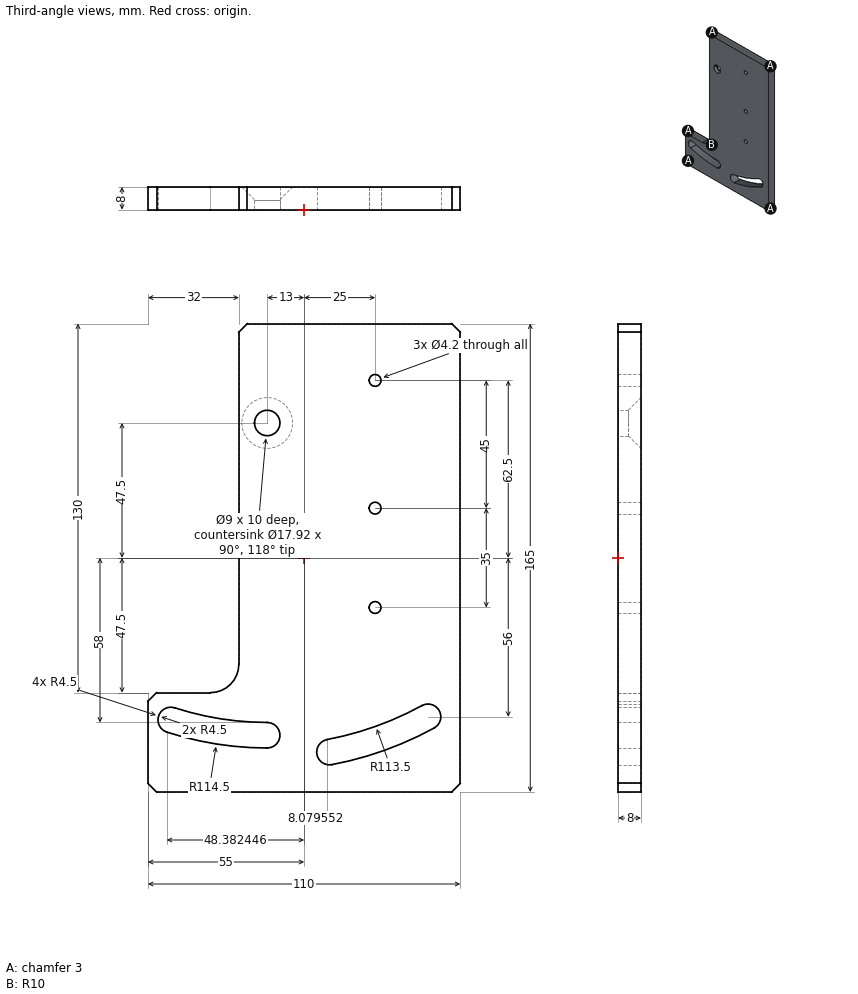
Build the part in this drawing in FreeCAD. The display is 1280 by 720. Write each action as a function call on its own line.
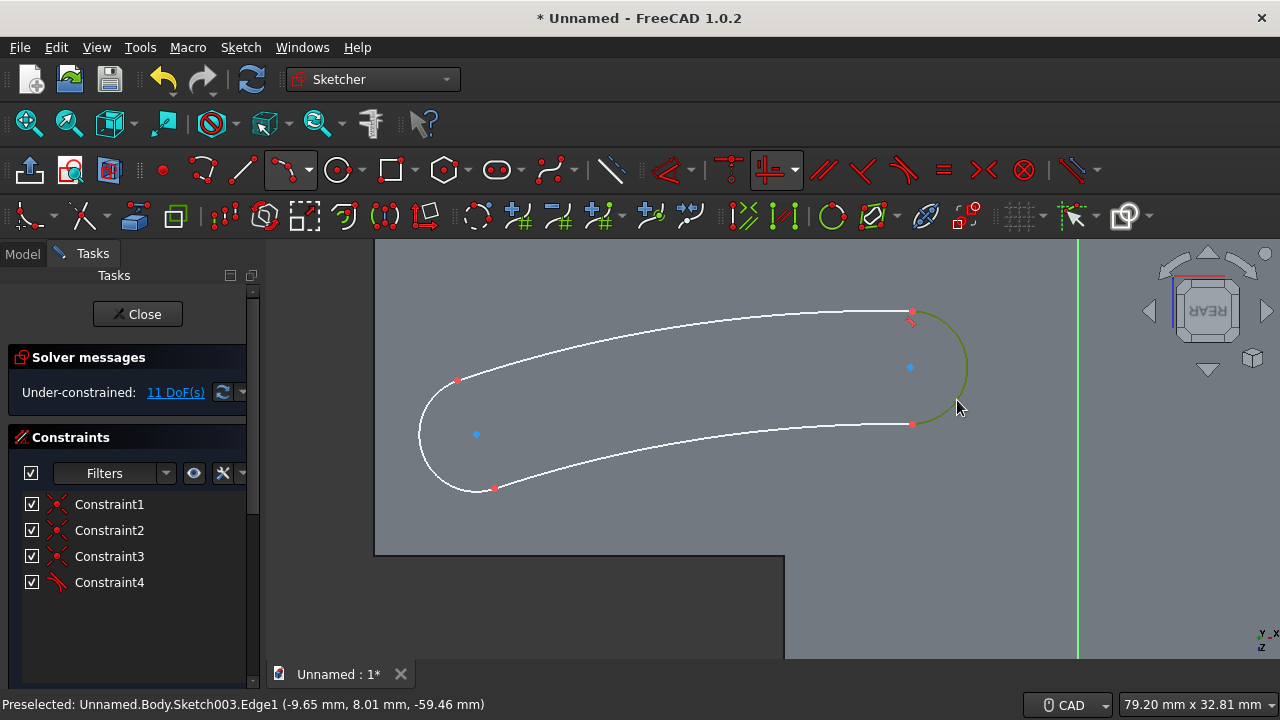
click(785, 429)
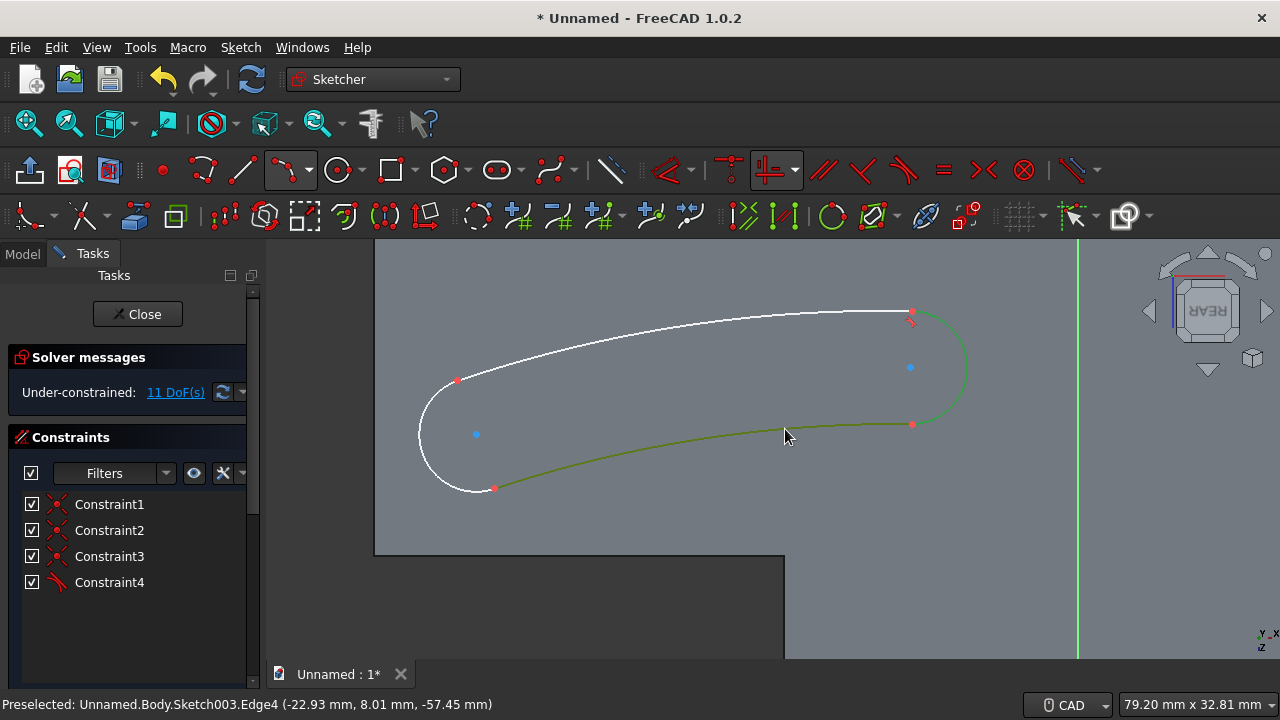
click(904, 170)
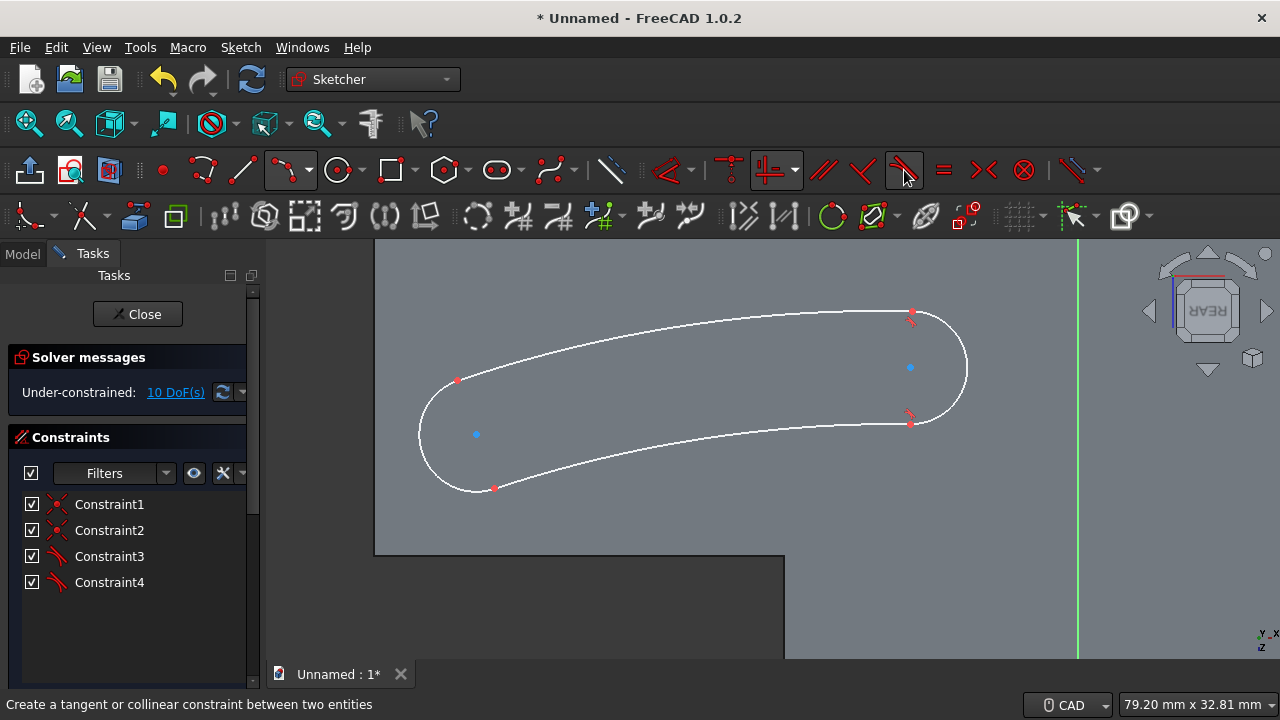
click(774, 315)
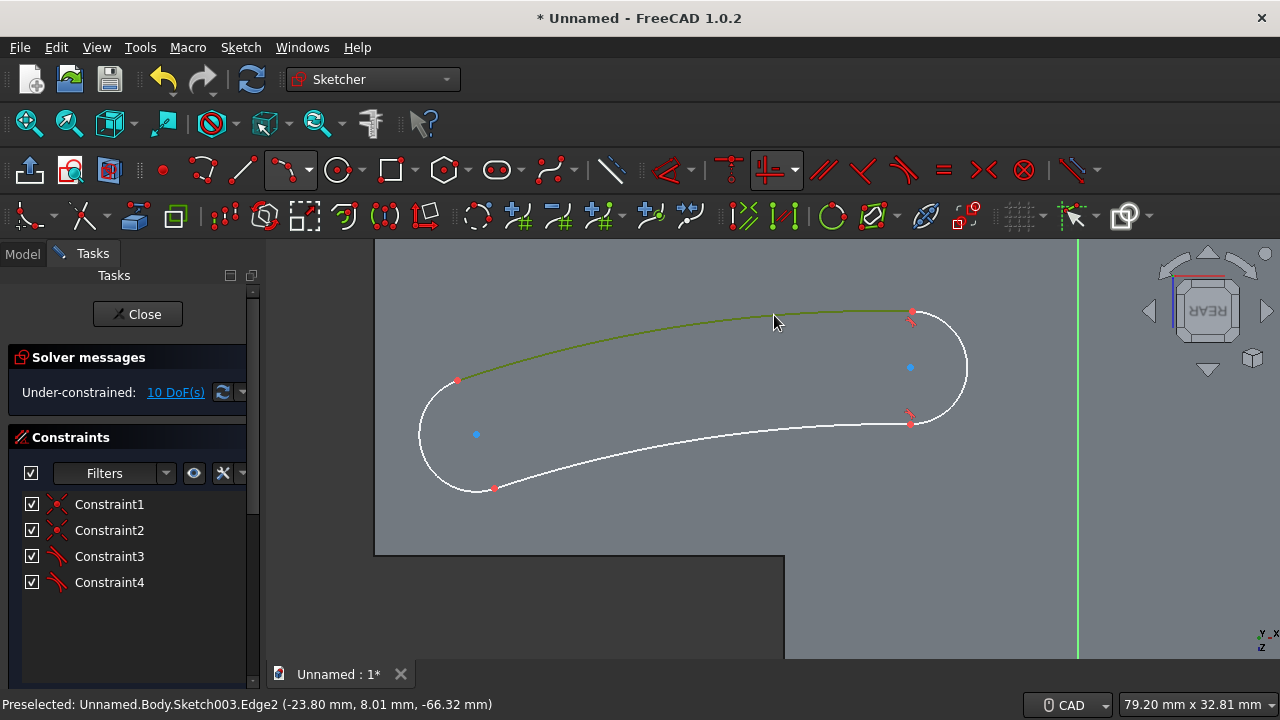
click(422, 418)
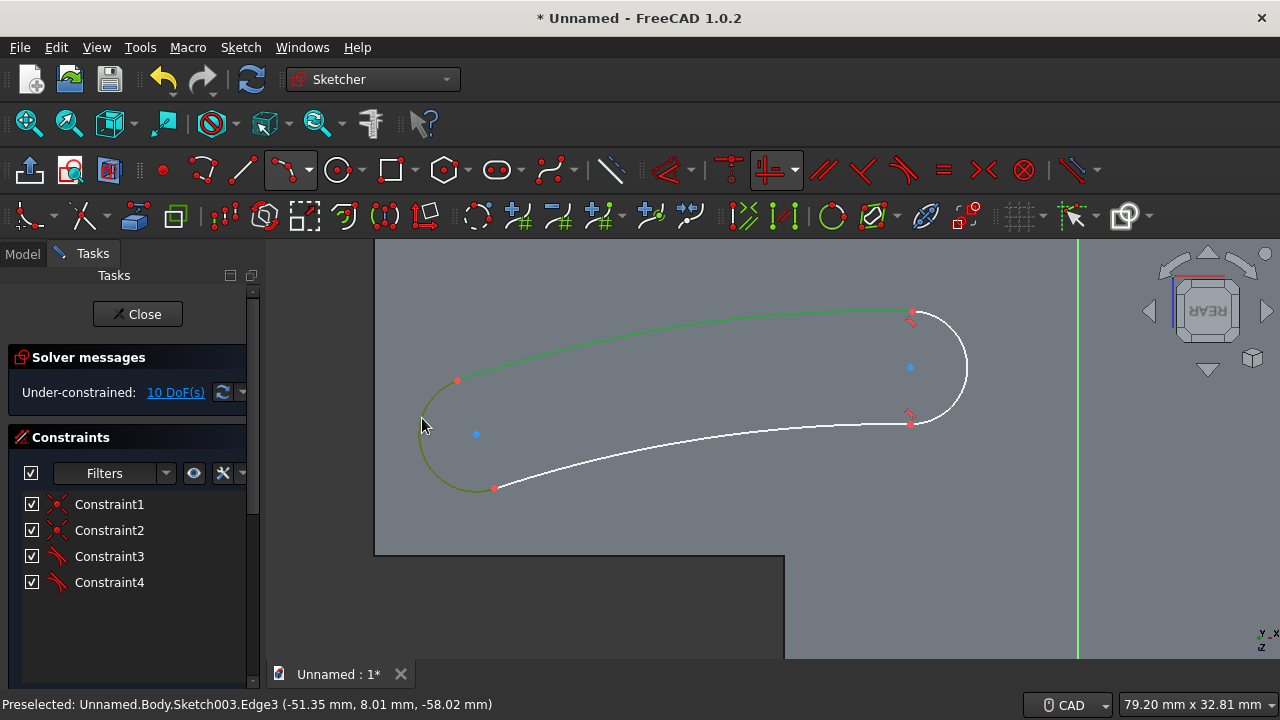
click(904, 170)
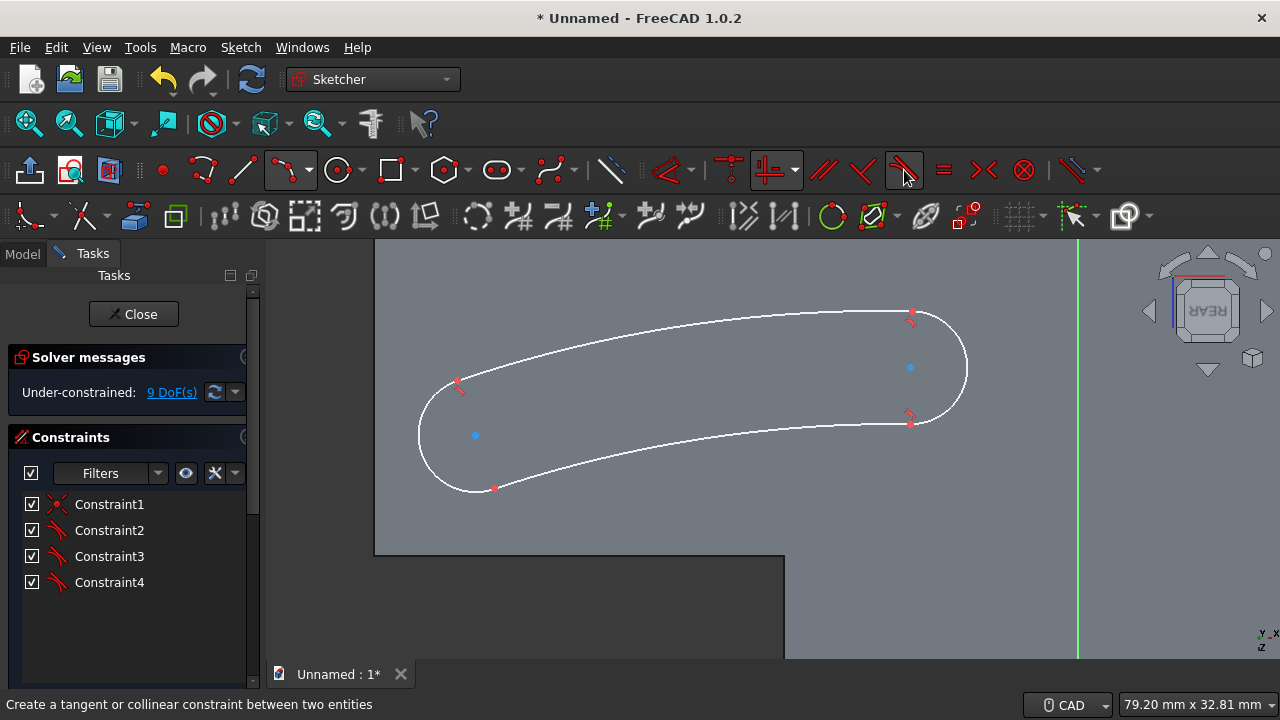
click(421, 418)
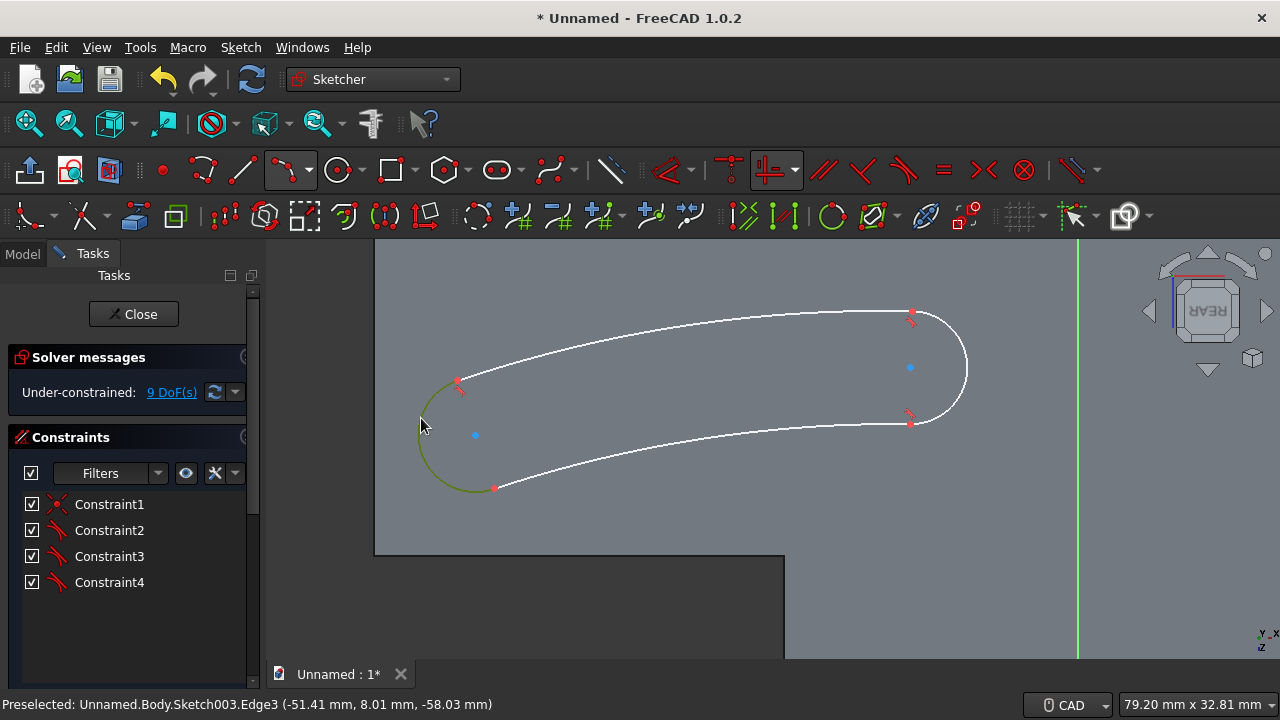
click(783, 429)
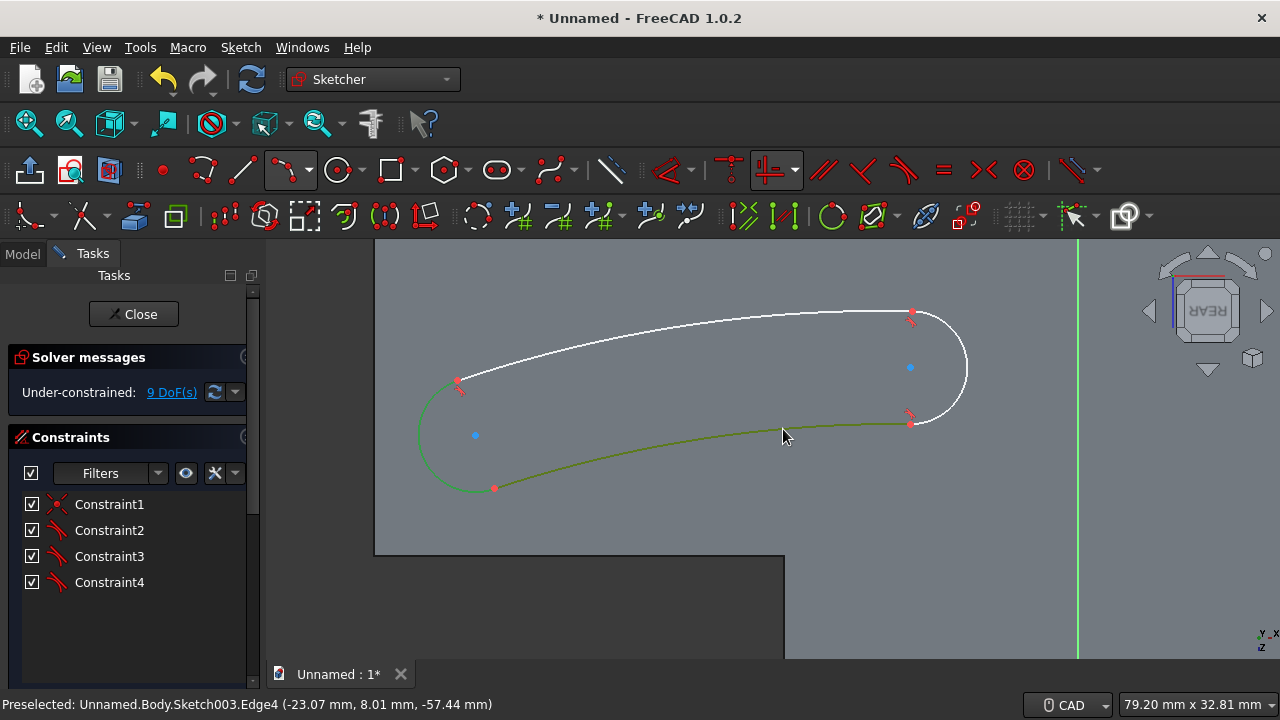
click(904, 170)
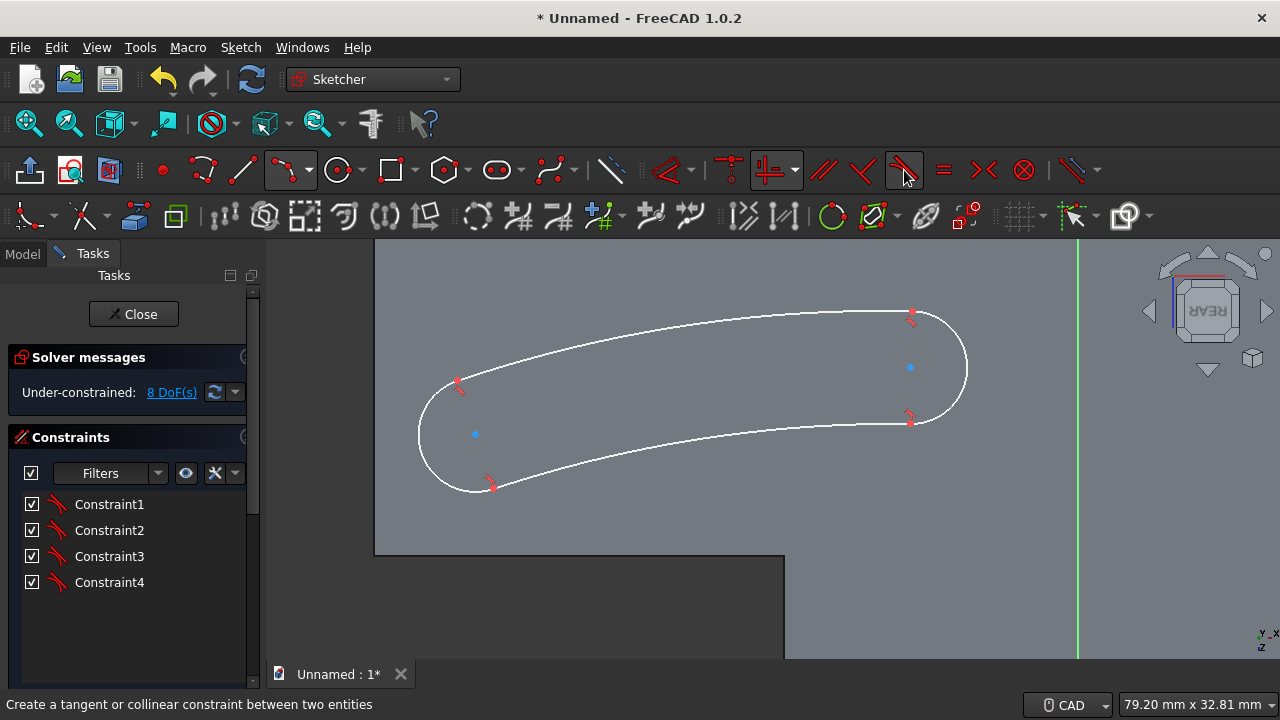
click(774, 315)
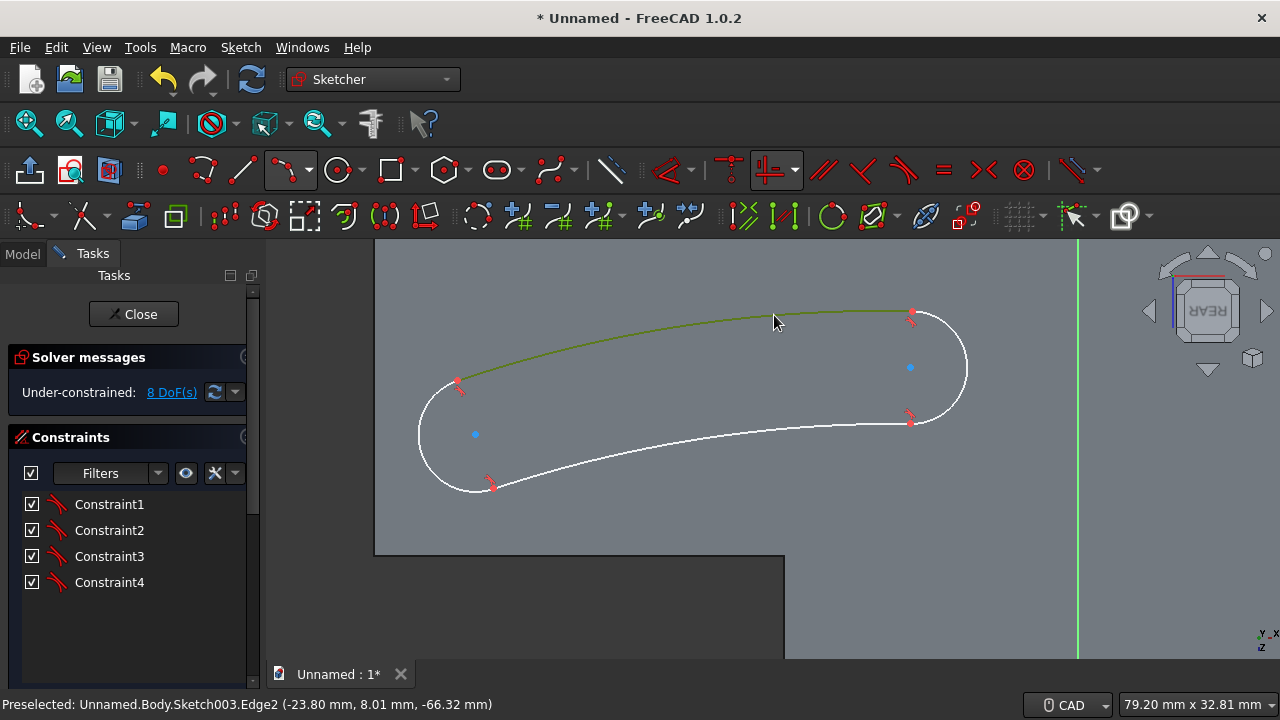
click(783, 429)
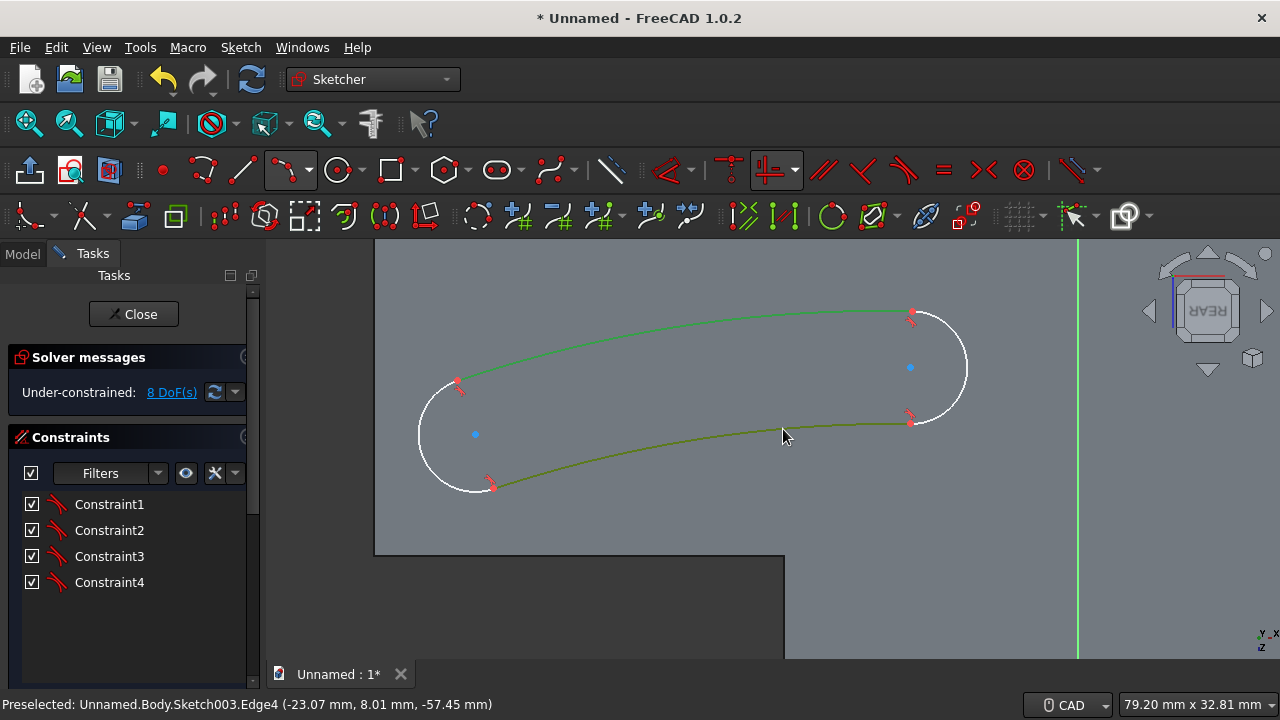
click(730, 170)